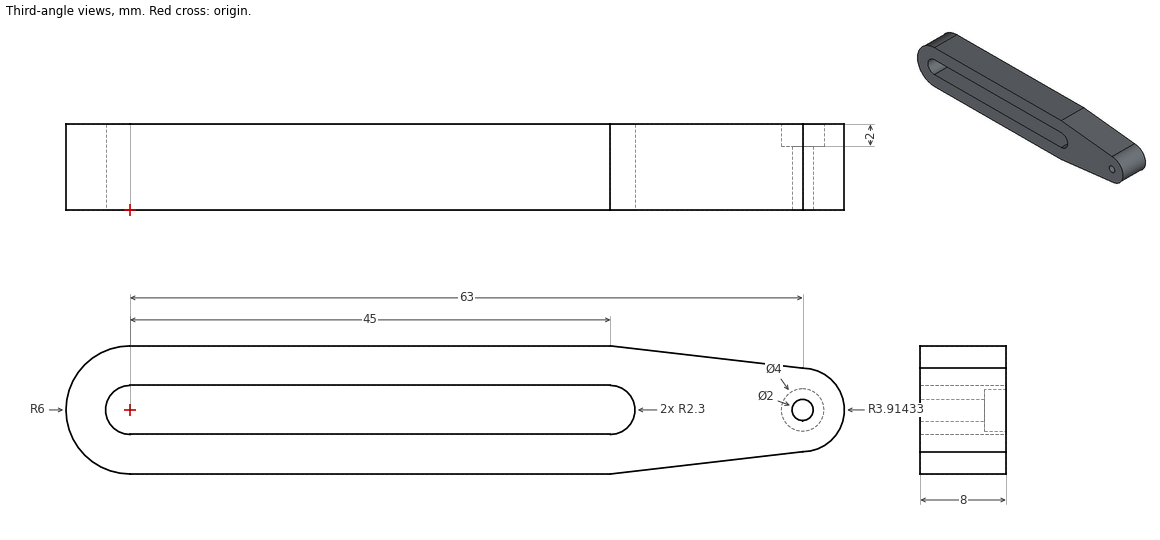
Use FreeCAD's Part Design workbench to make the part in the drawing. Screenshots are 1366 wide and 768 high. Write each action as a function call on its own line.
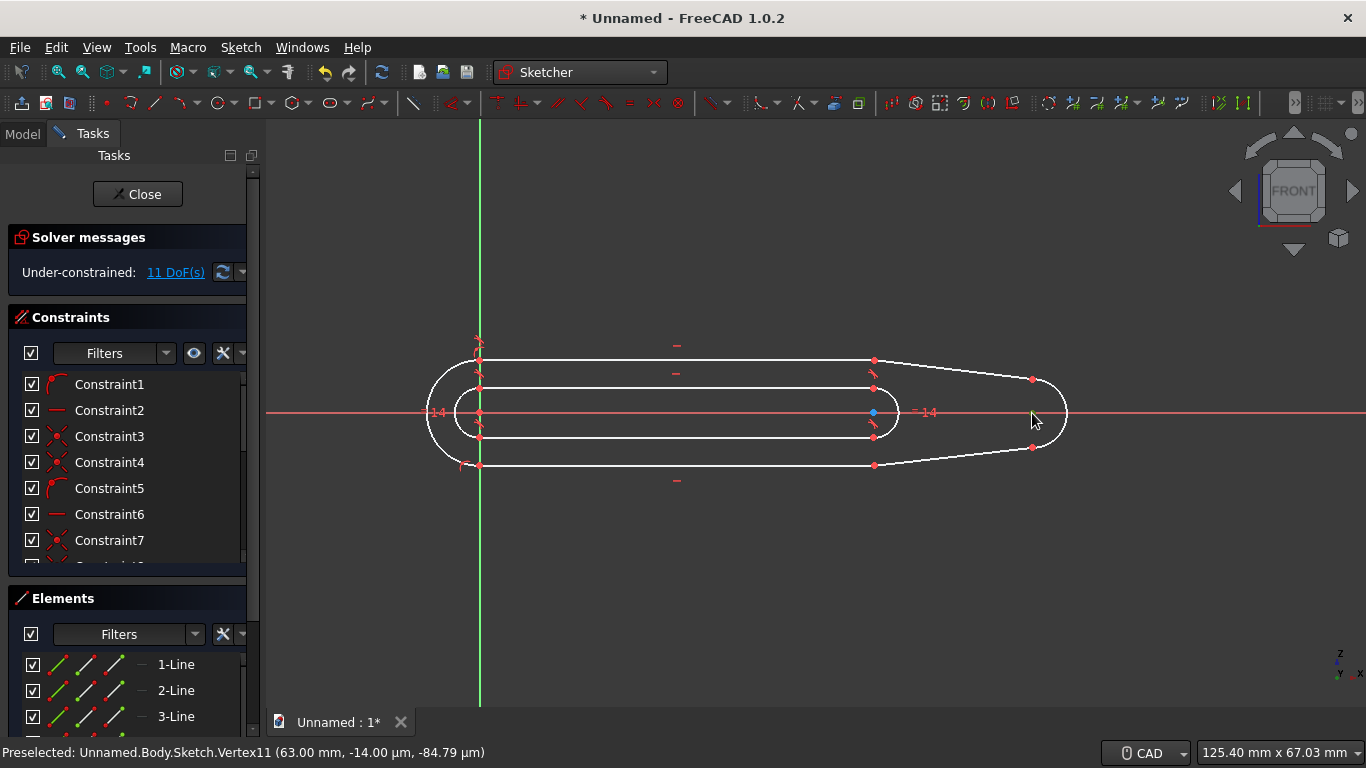
click(359, 413)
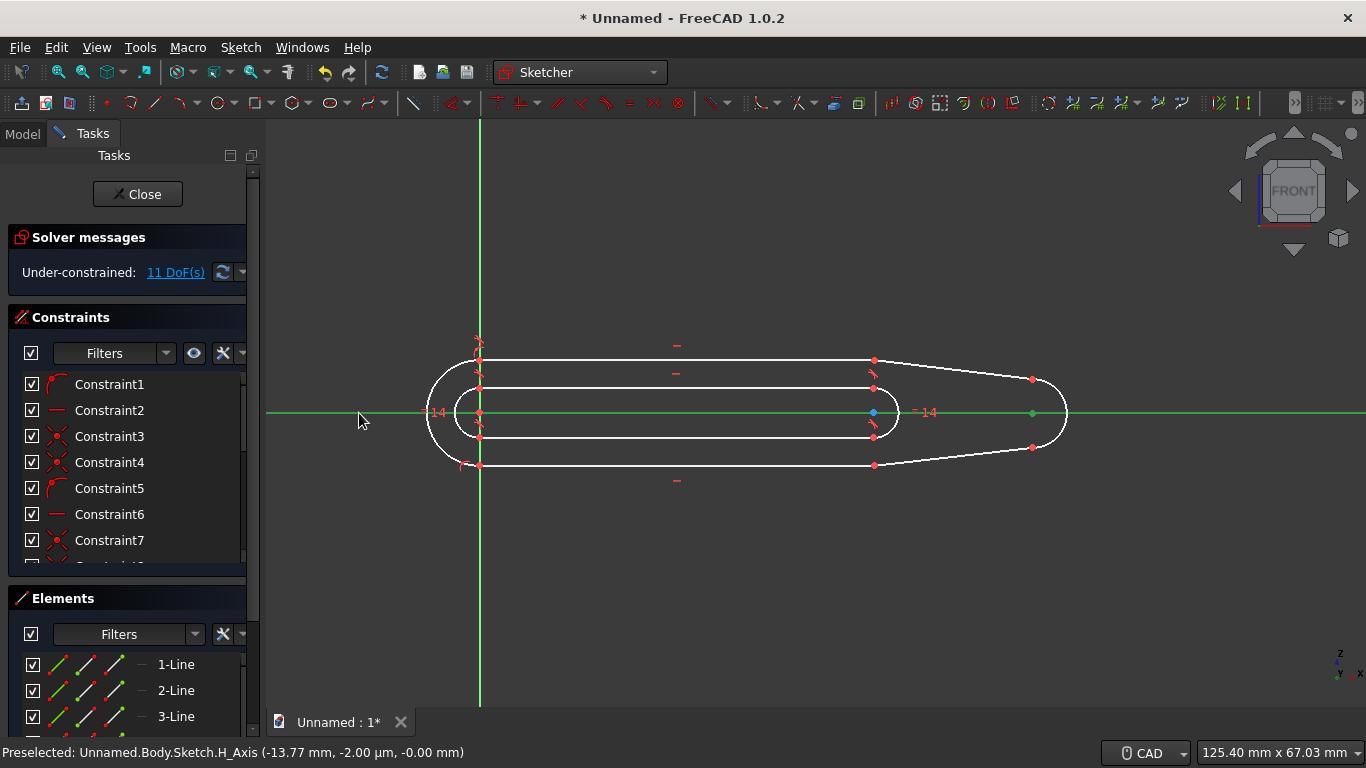
click(498, 104)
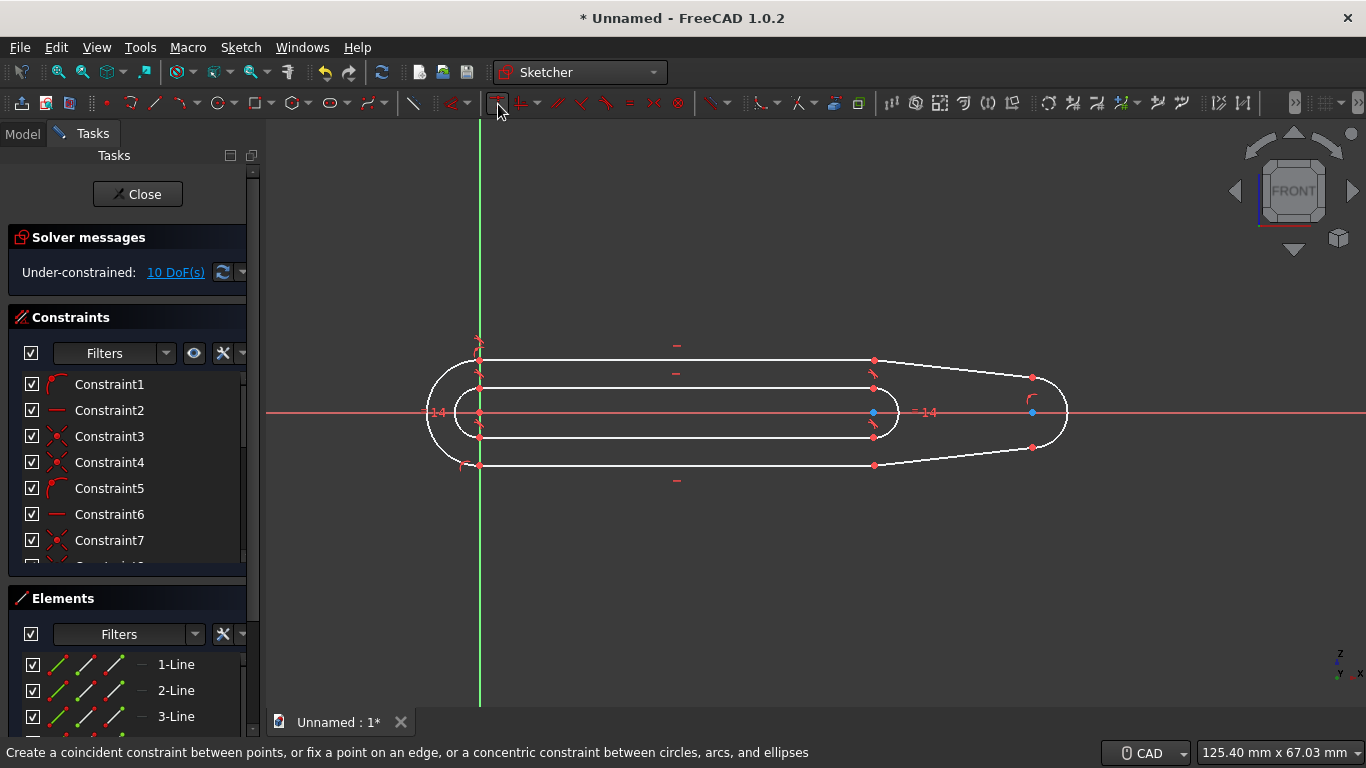
click(480, 413)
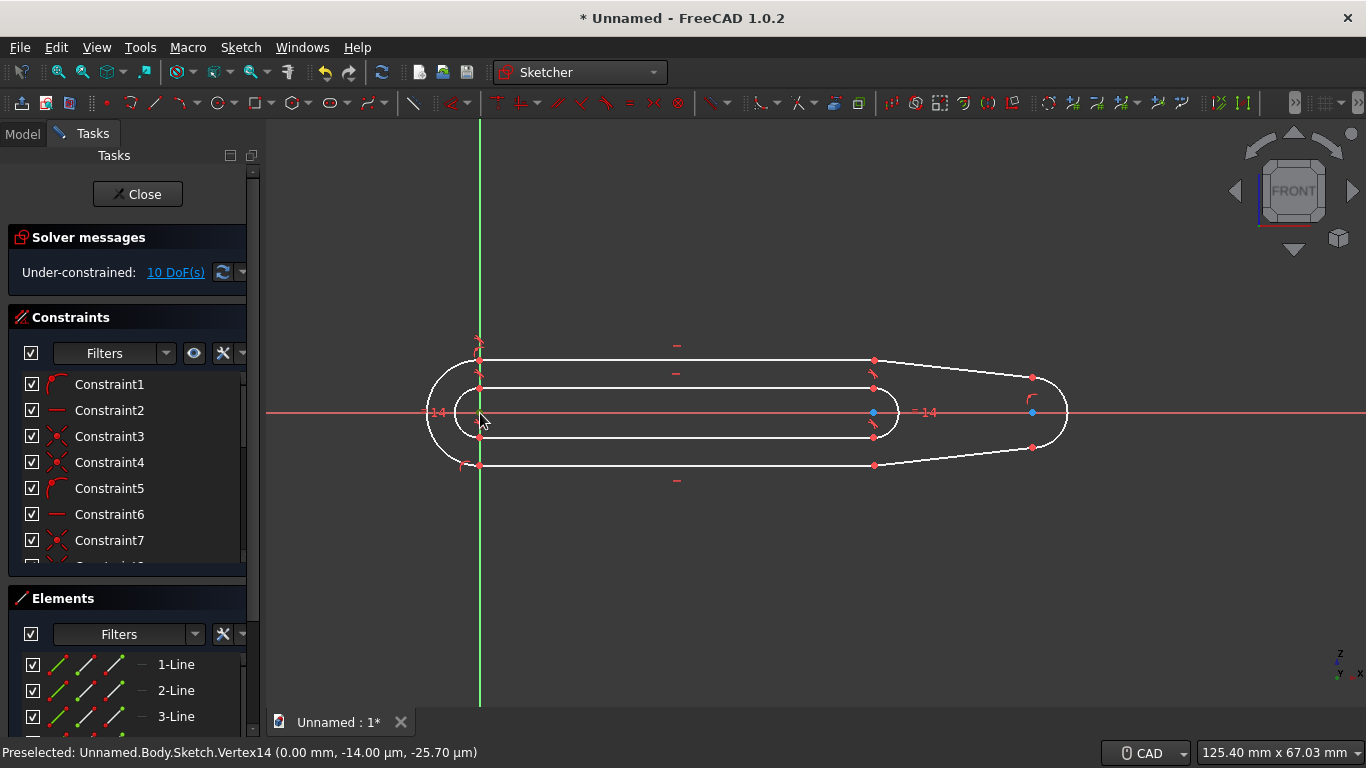
click(359, 413)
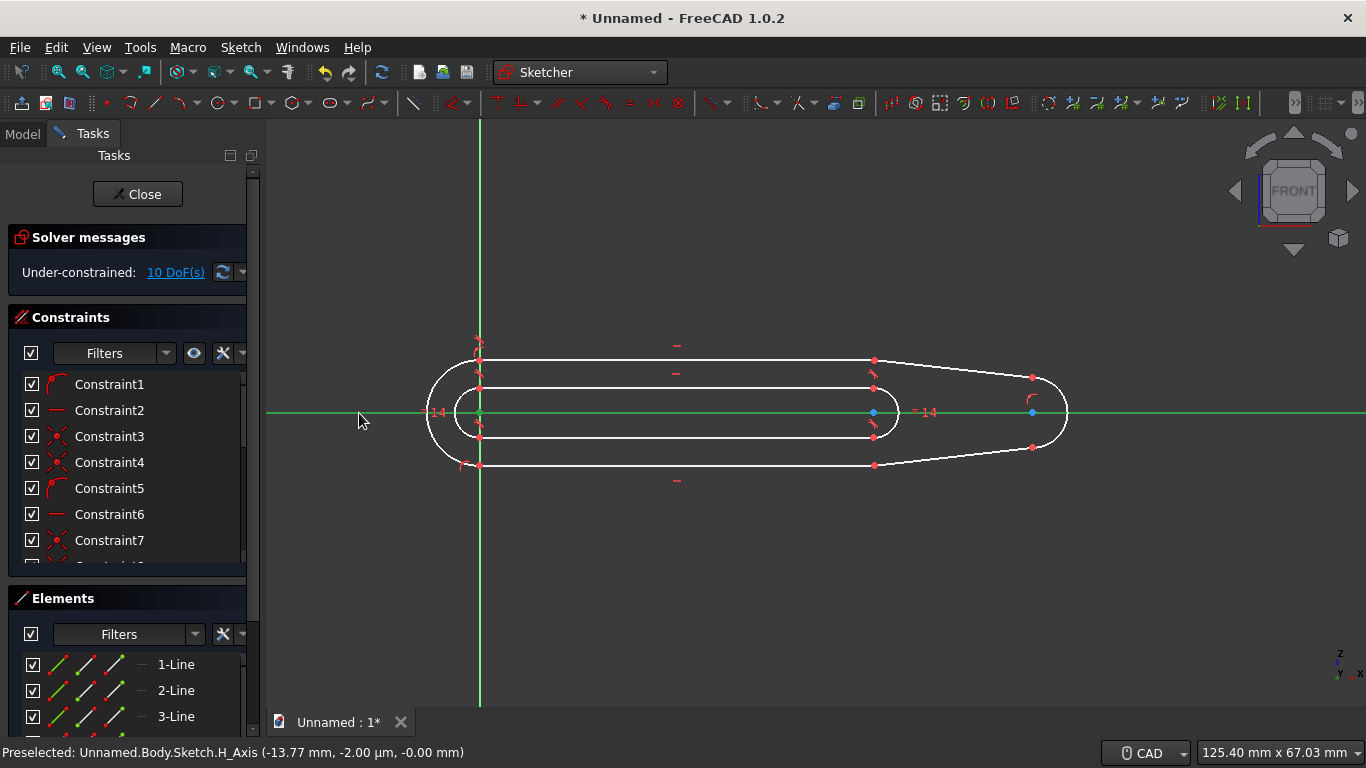
click(498, 104)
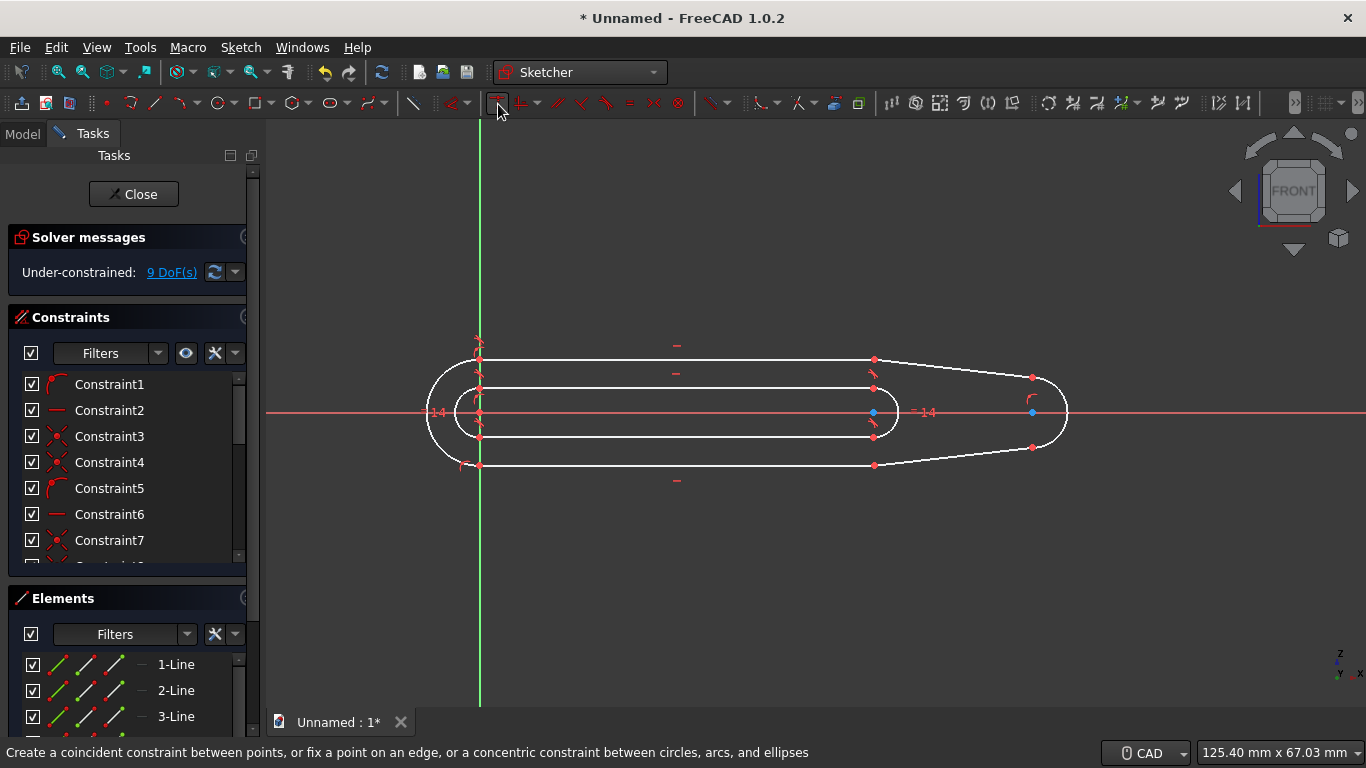
click(1061, 433)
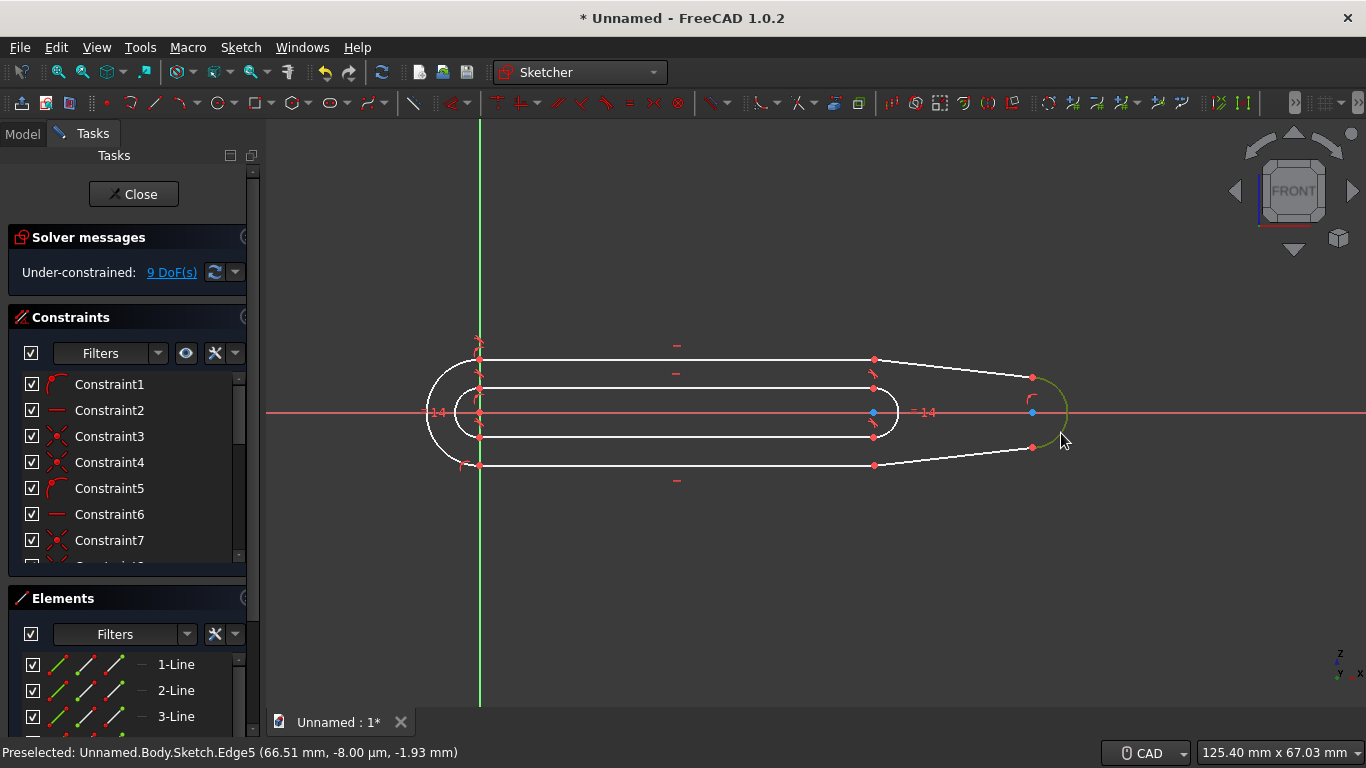
key(k)
key(r)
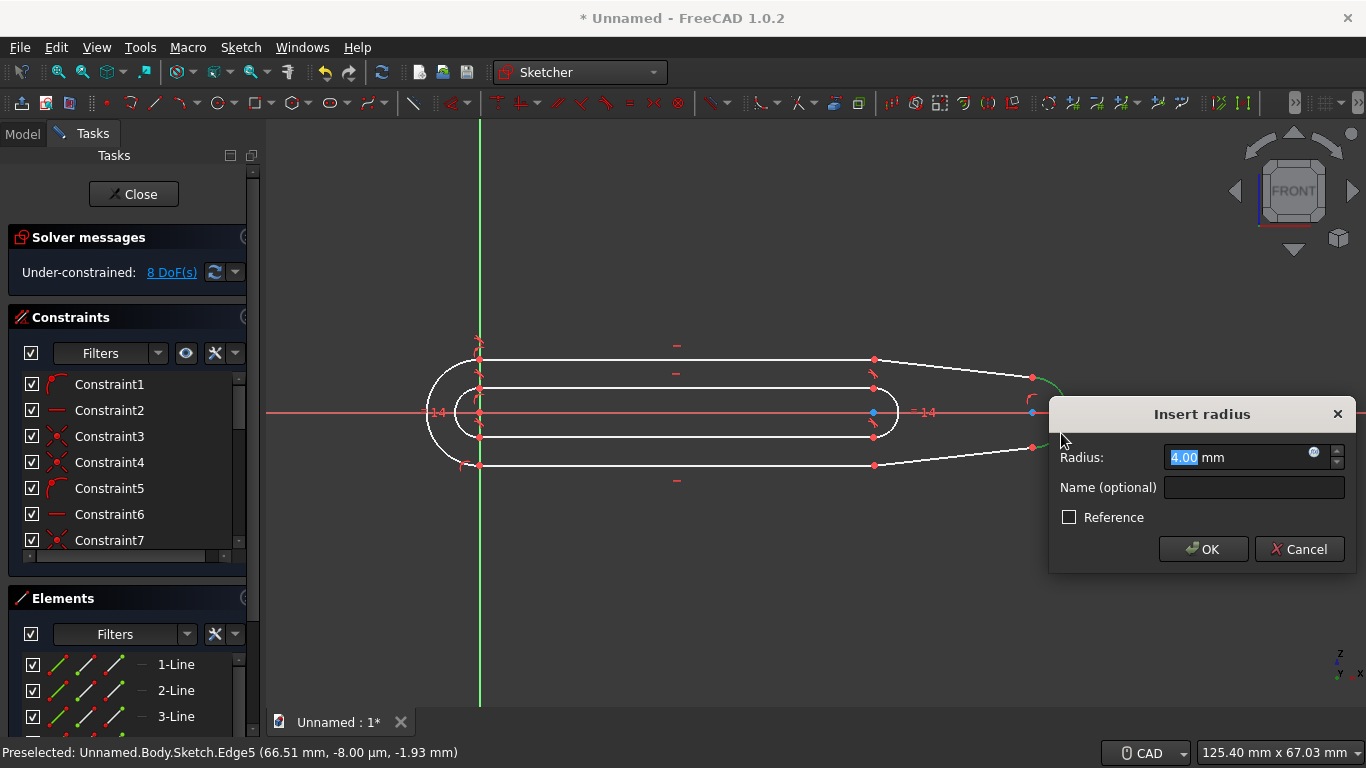
text(3.91433)
key(Return)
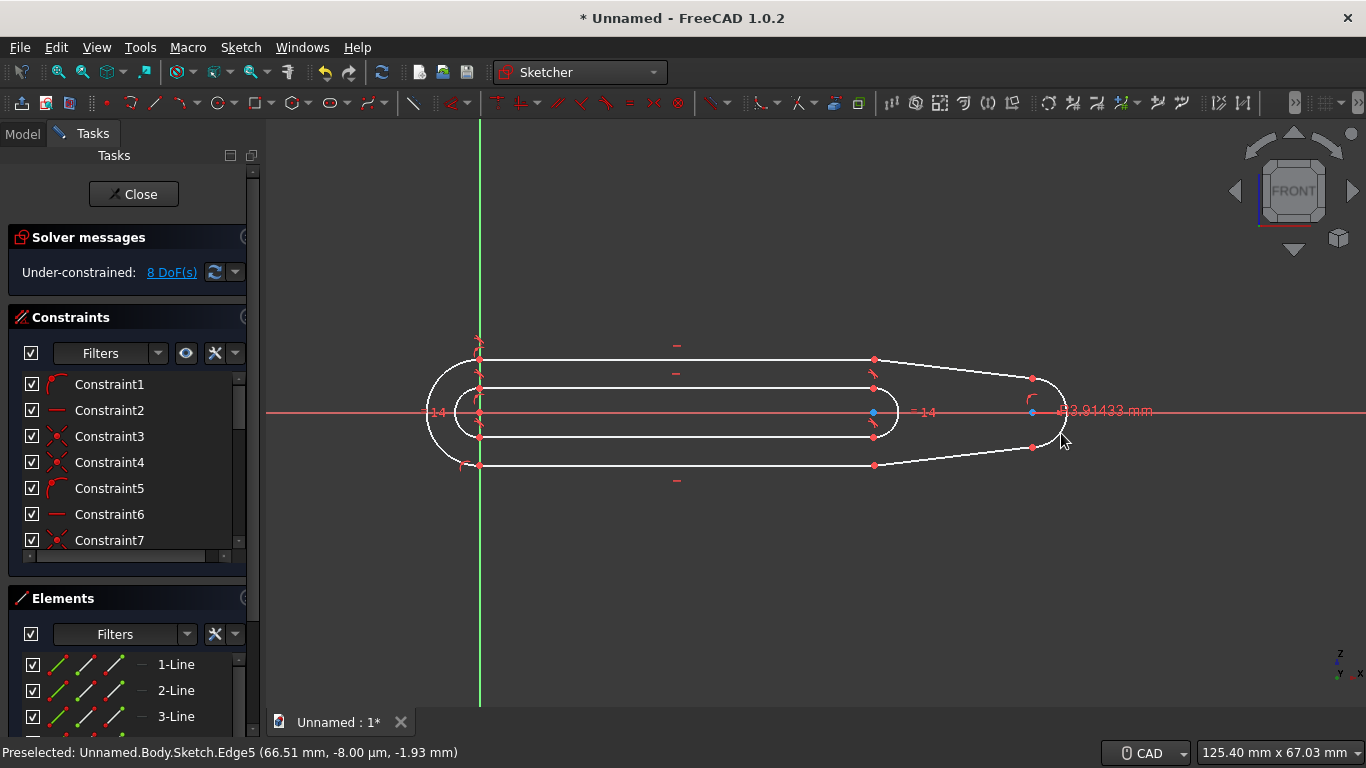
click(437, 382)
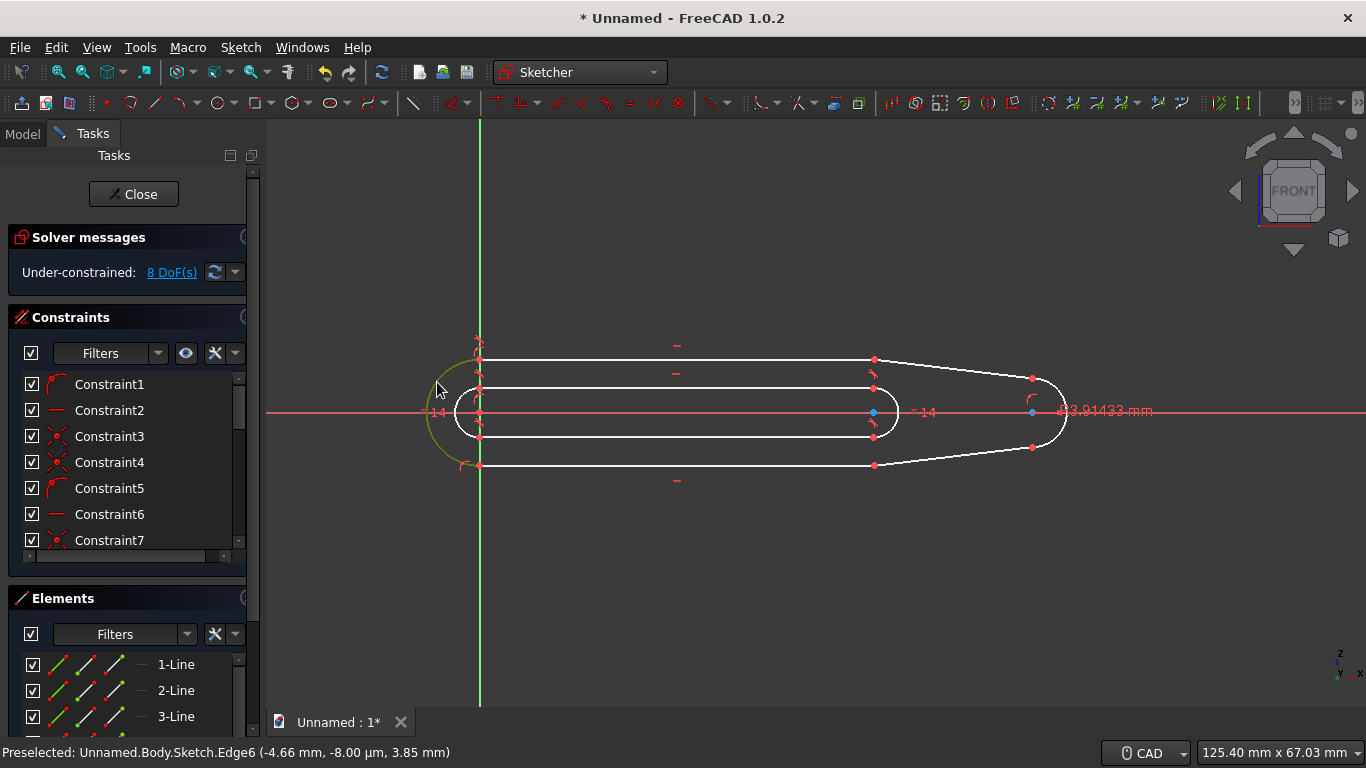
click(470, 104)